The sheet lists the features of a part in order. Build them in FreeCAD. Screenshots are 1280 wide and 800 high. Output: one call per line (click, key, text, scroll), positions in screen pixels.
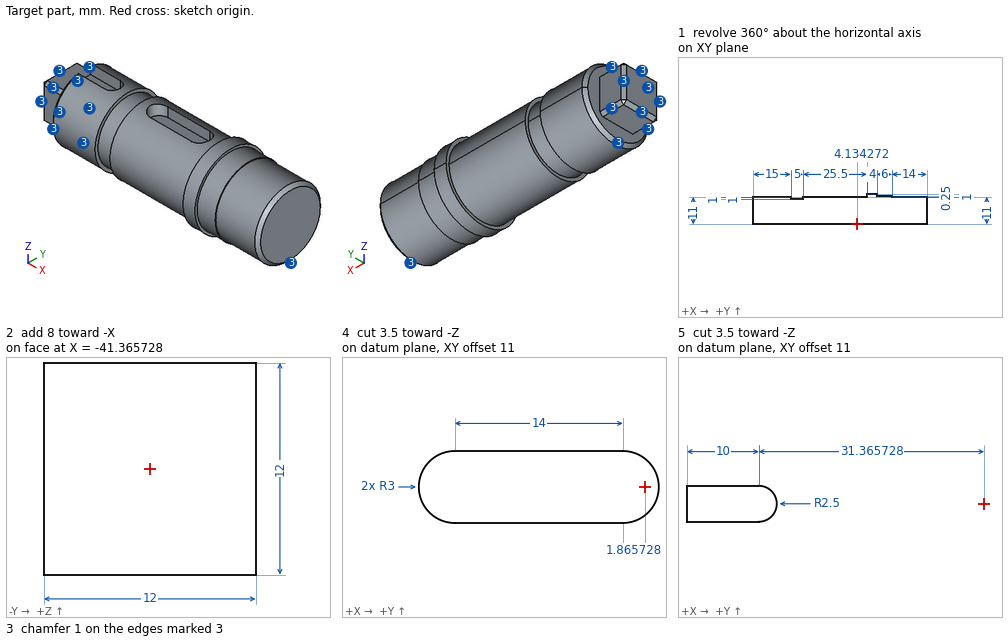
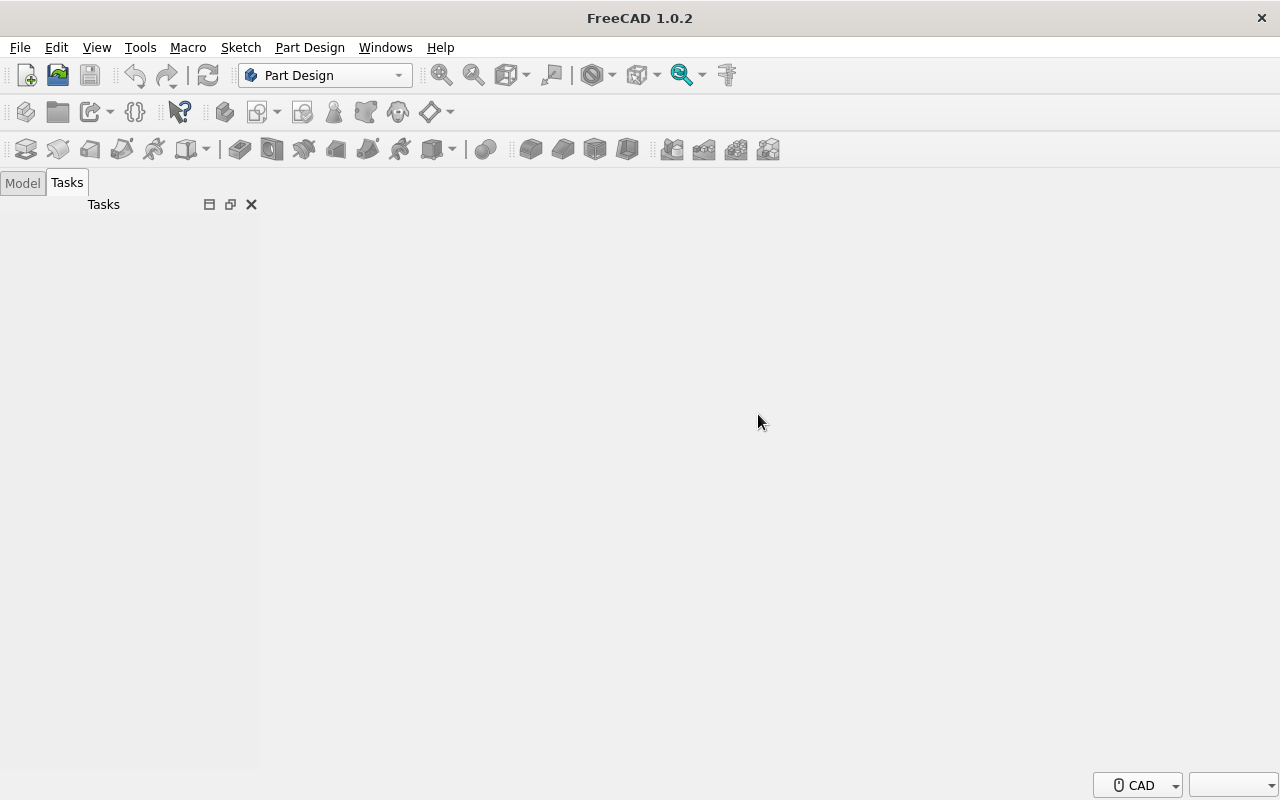
click(26, 76)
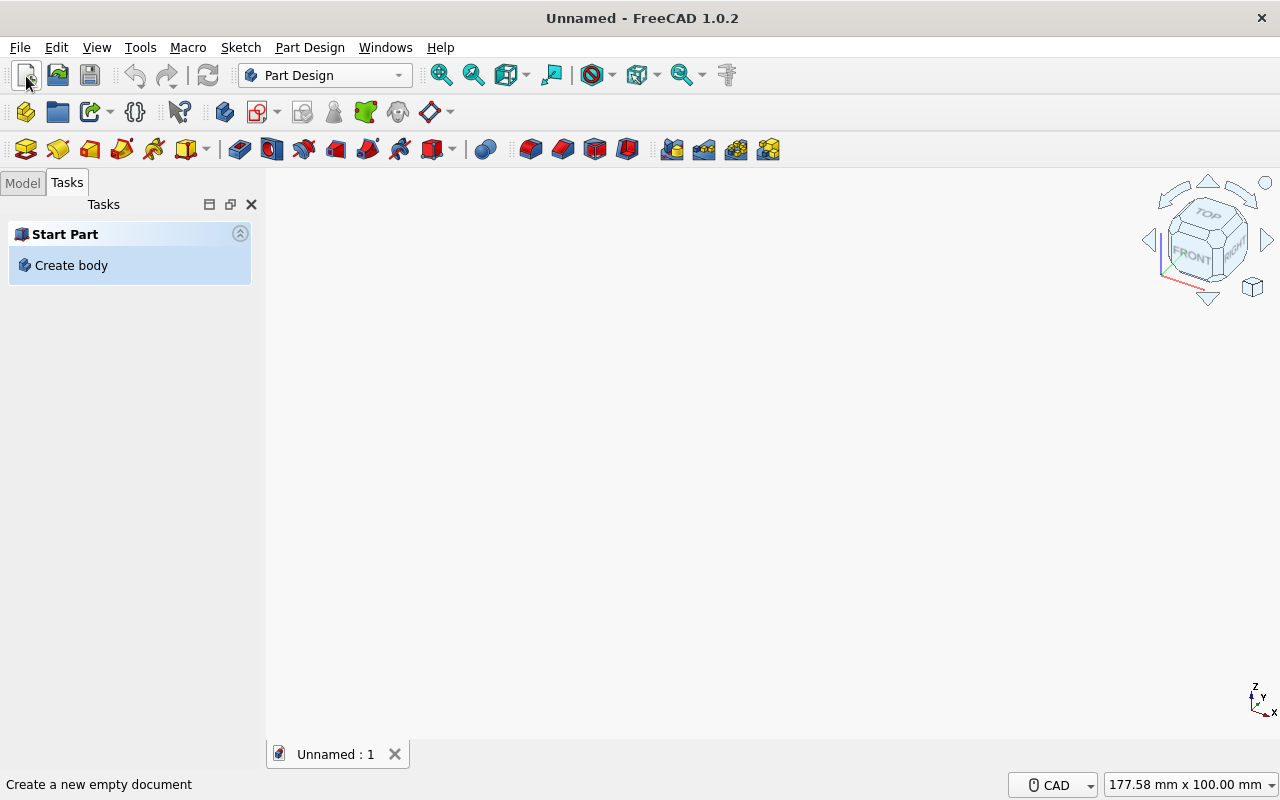
click(258, 112)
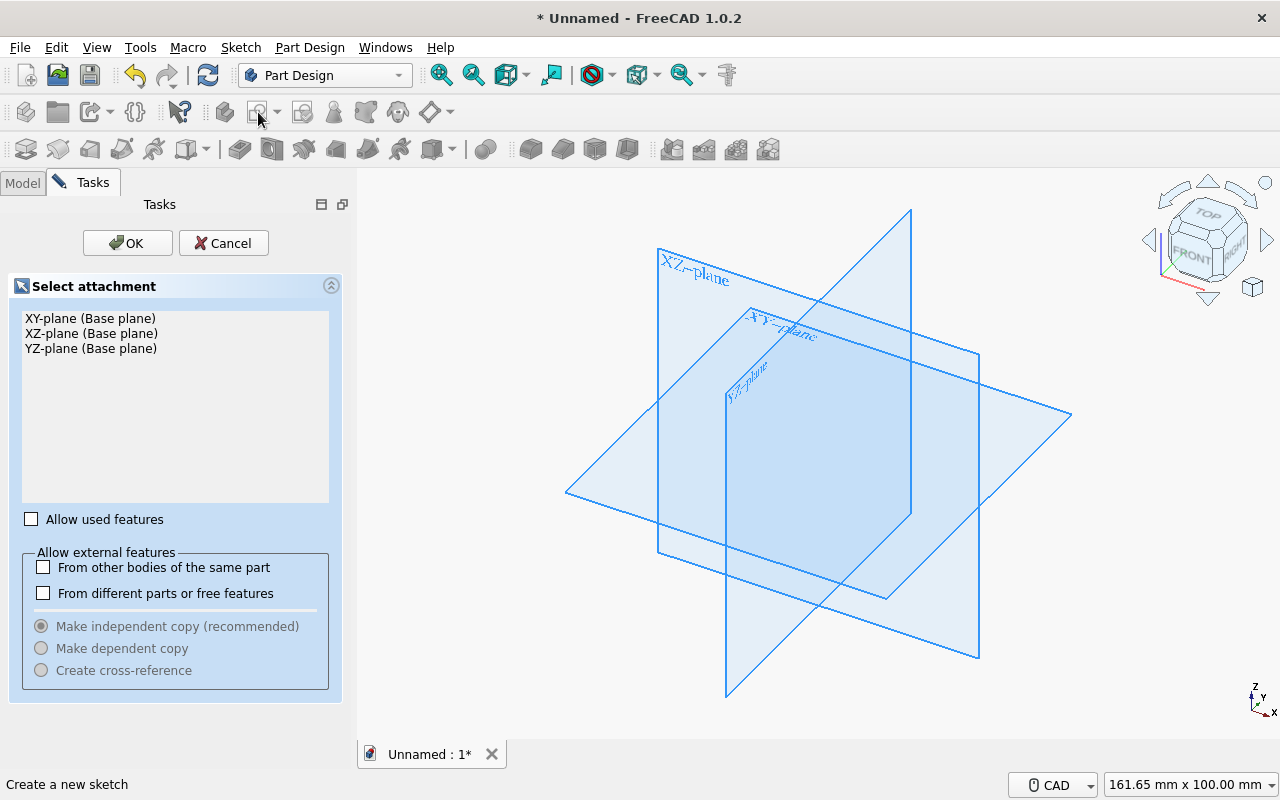
click(82, 318)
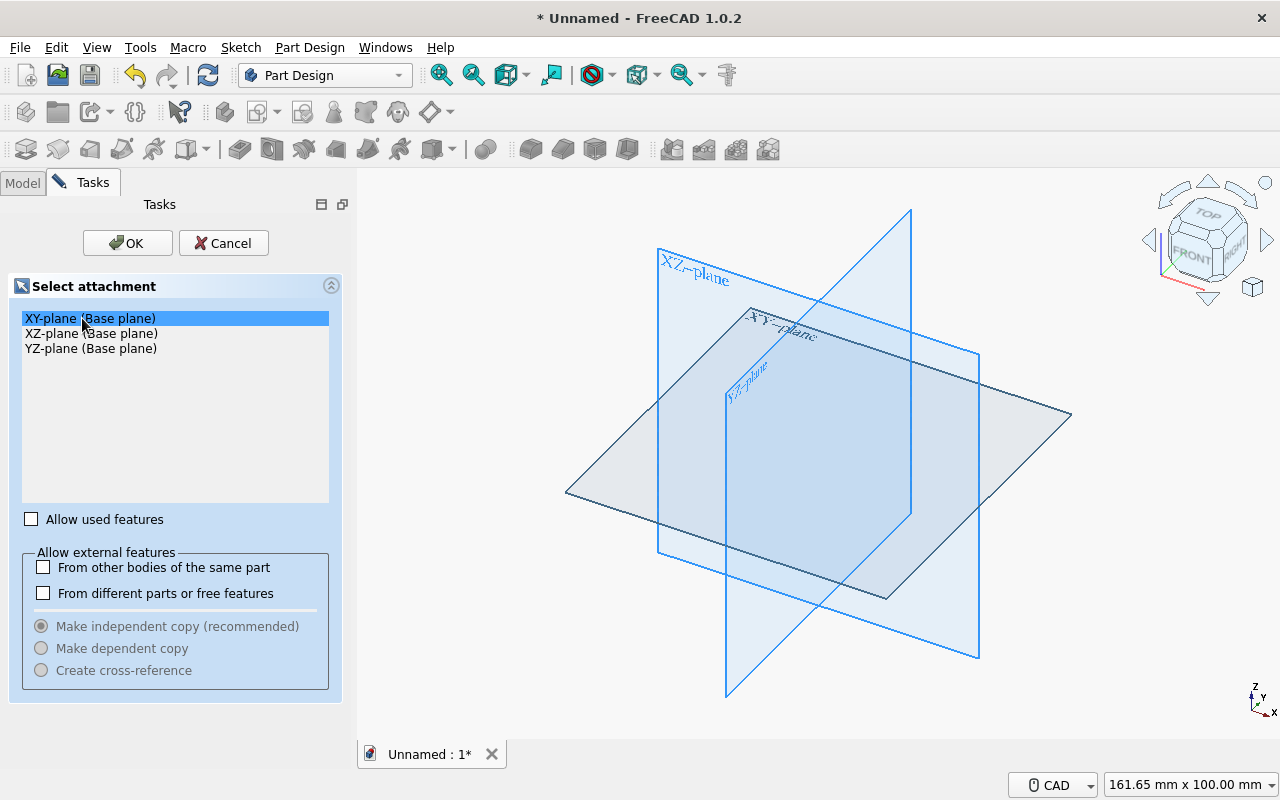
click(128, 243)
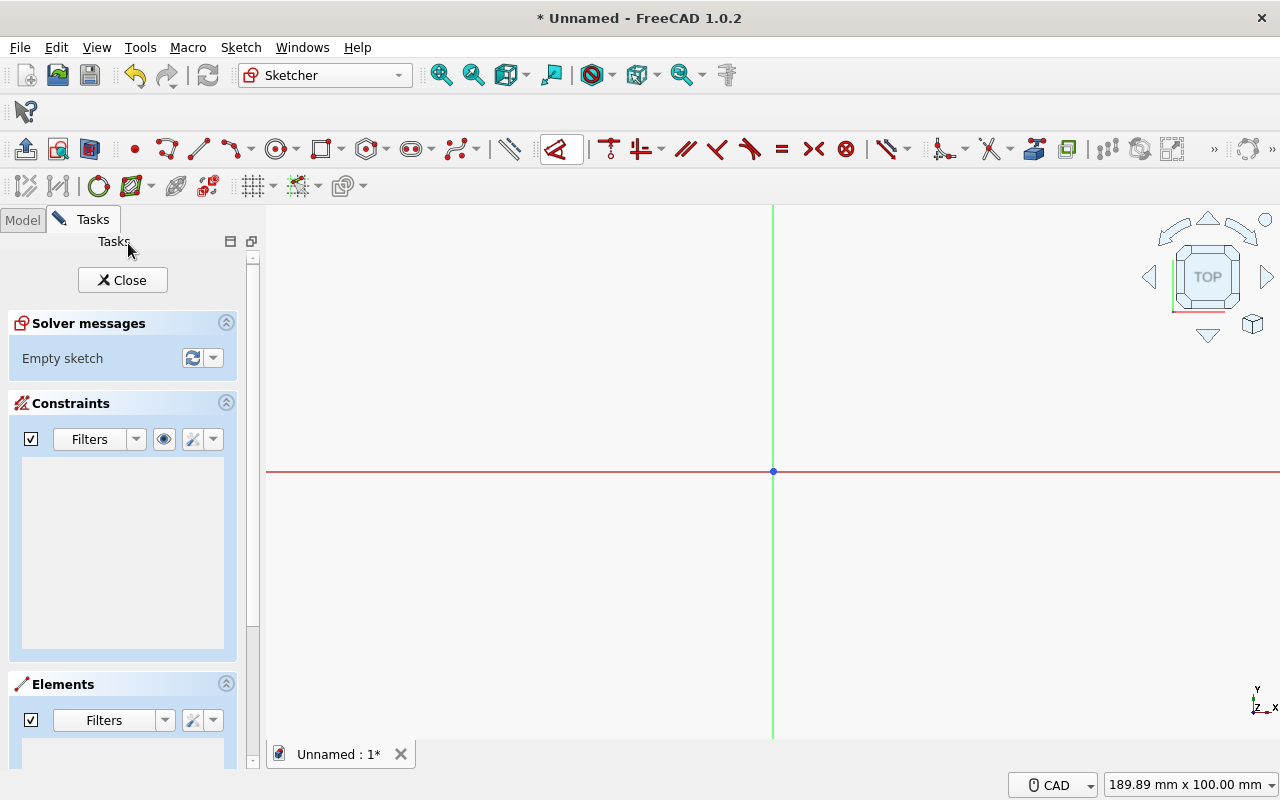
scroll(805, 375, up, 2)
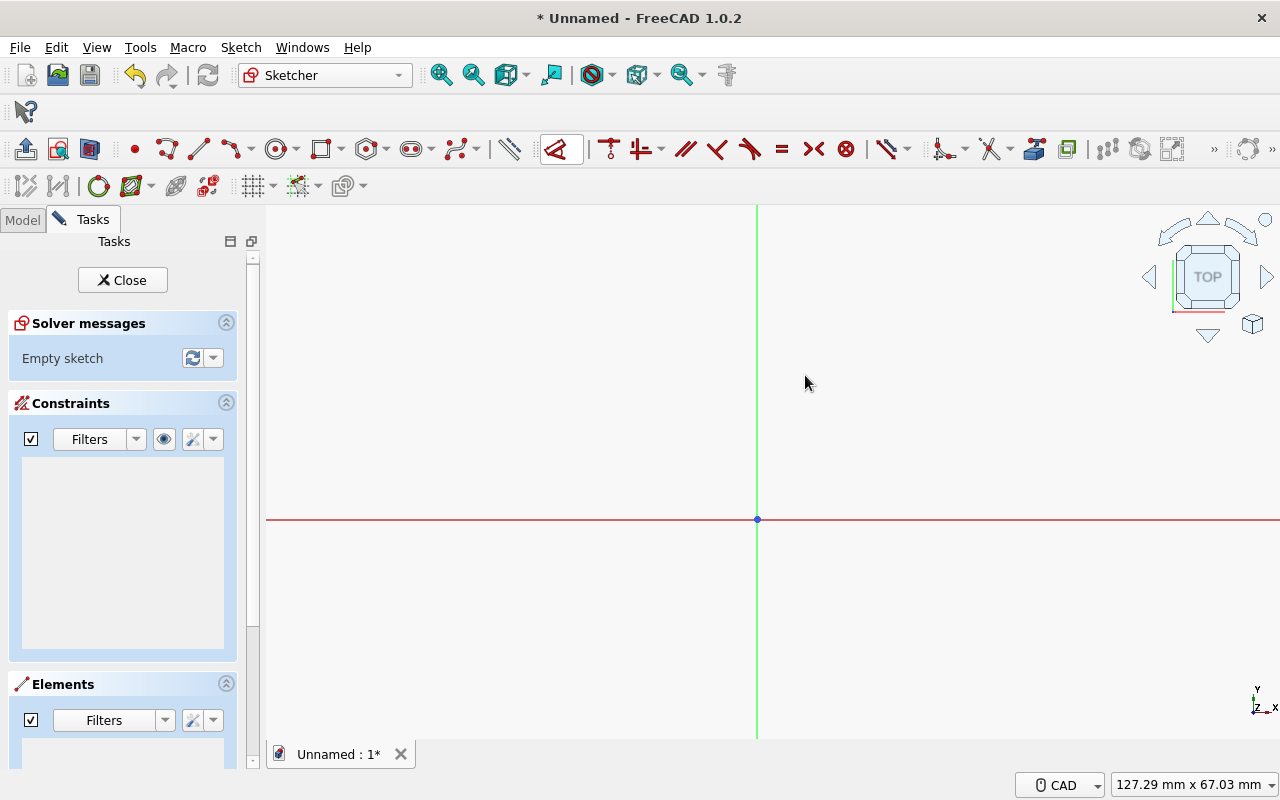
click(168, 150)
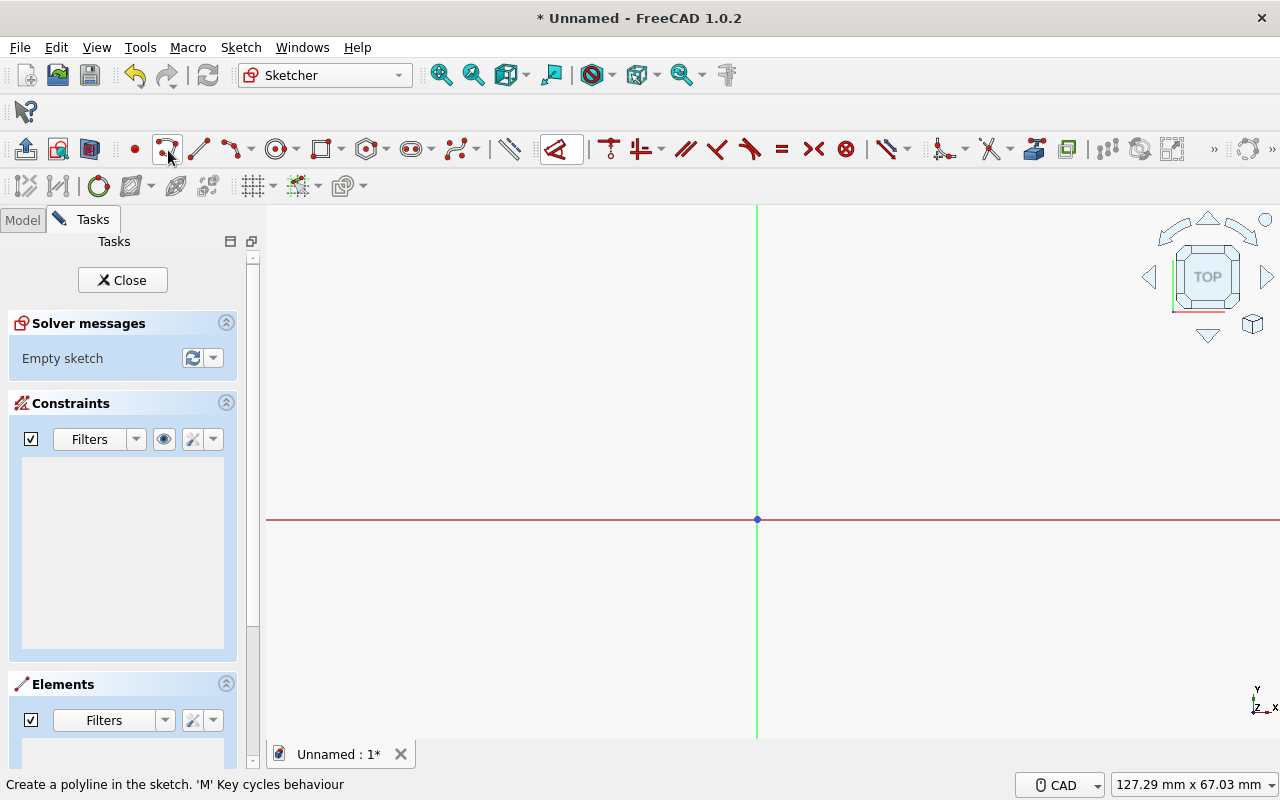
click(790, 432)
click(587, 432)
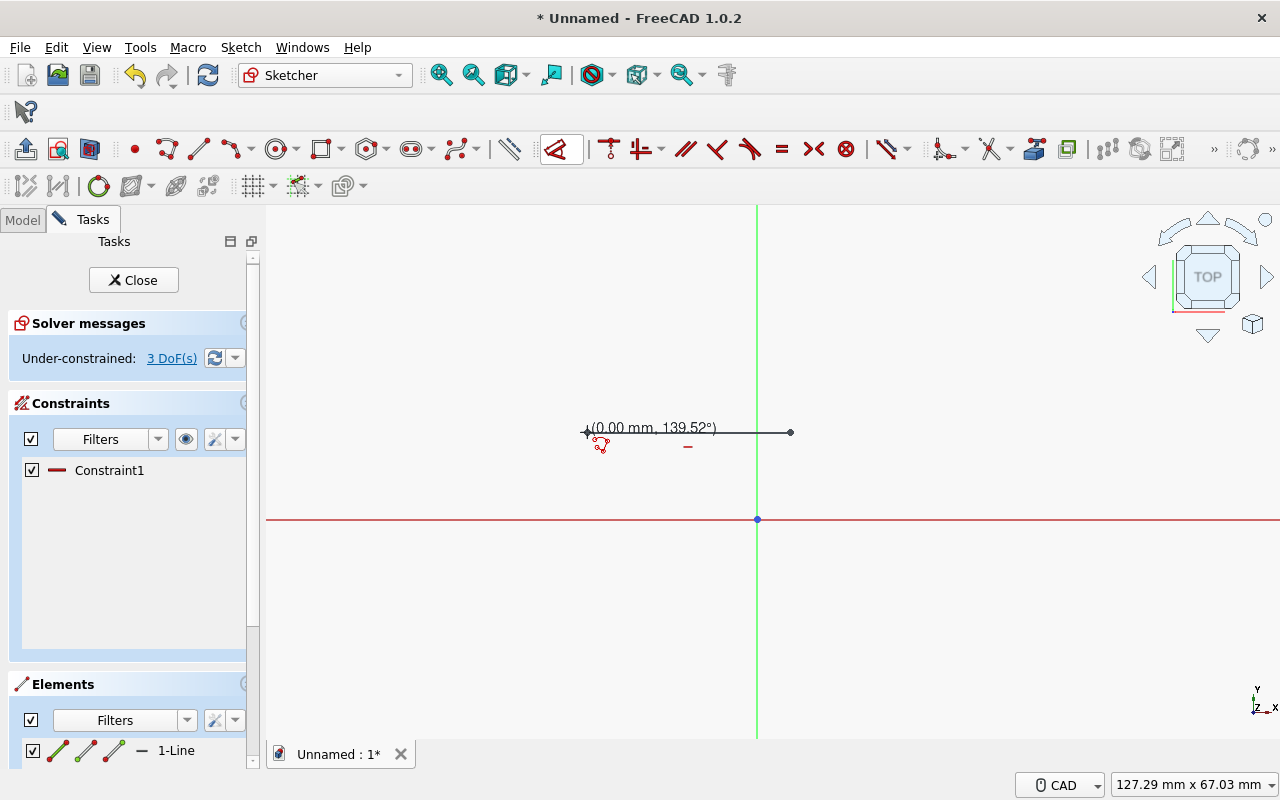
scroll(587, 440, up, 4)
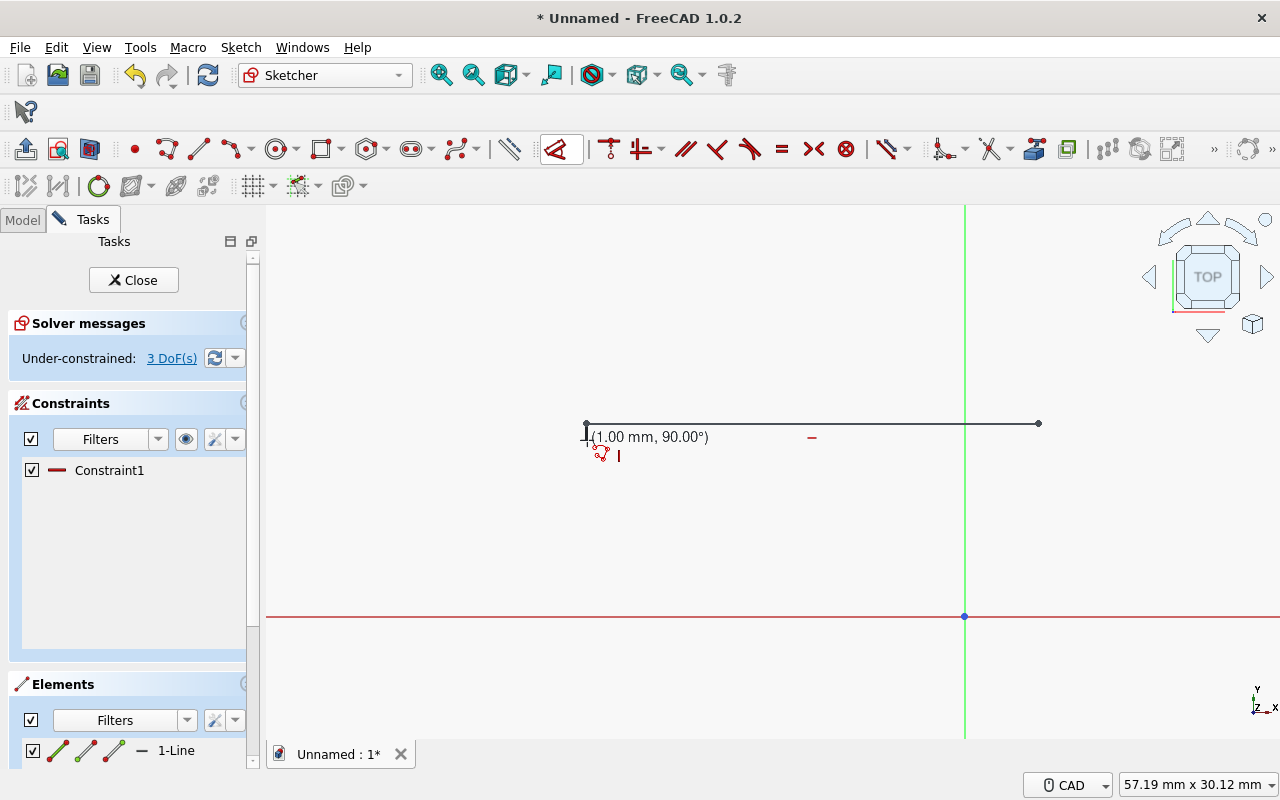
click(587, 439)
click(498, 439)
click(498, 421)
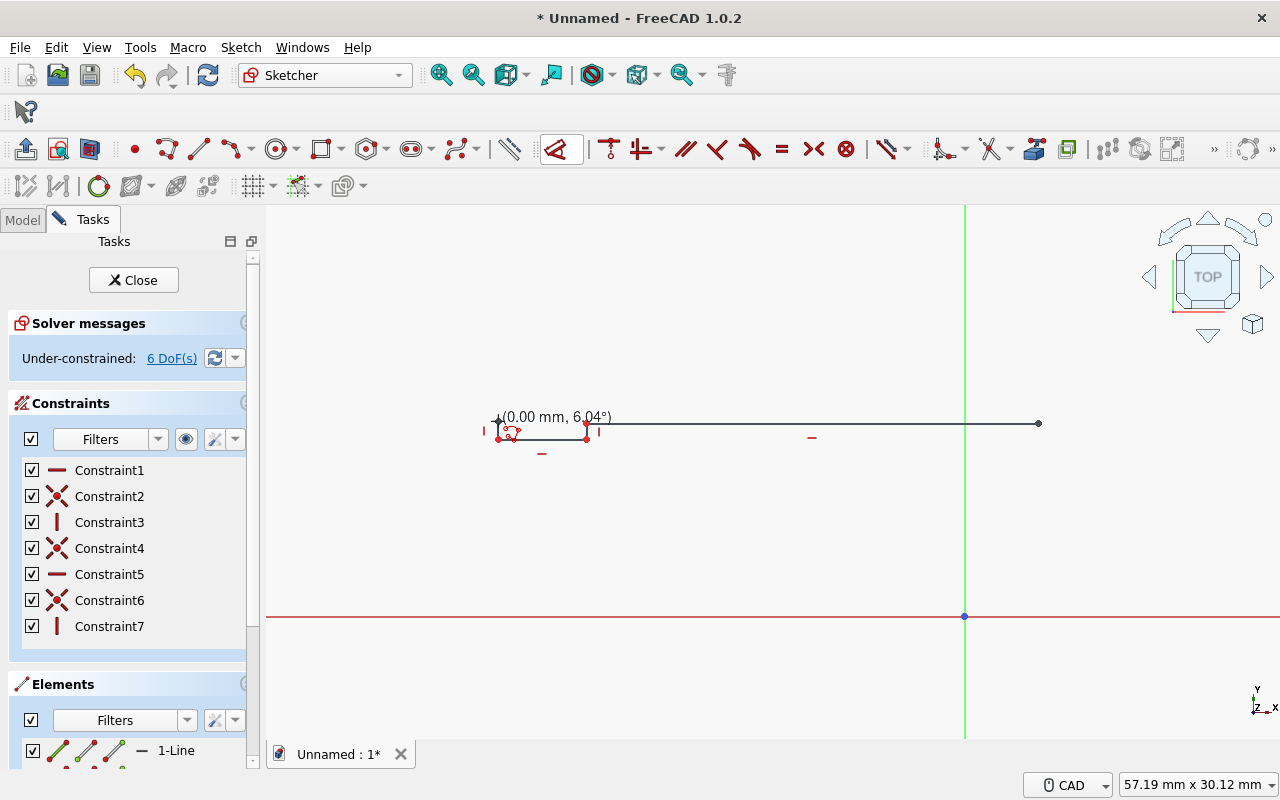
scroll(588, 441, down, 4)